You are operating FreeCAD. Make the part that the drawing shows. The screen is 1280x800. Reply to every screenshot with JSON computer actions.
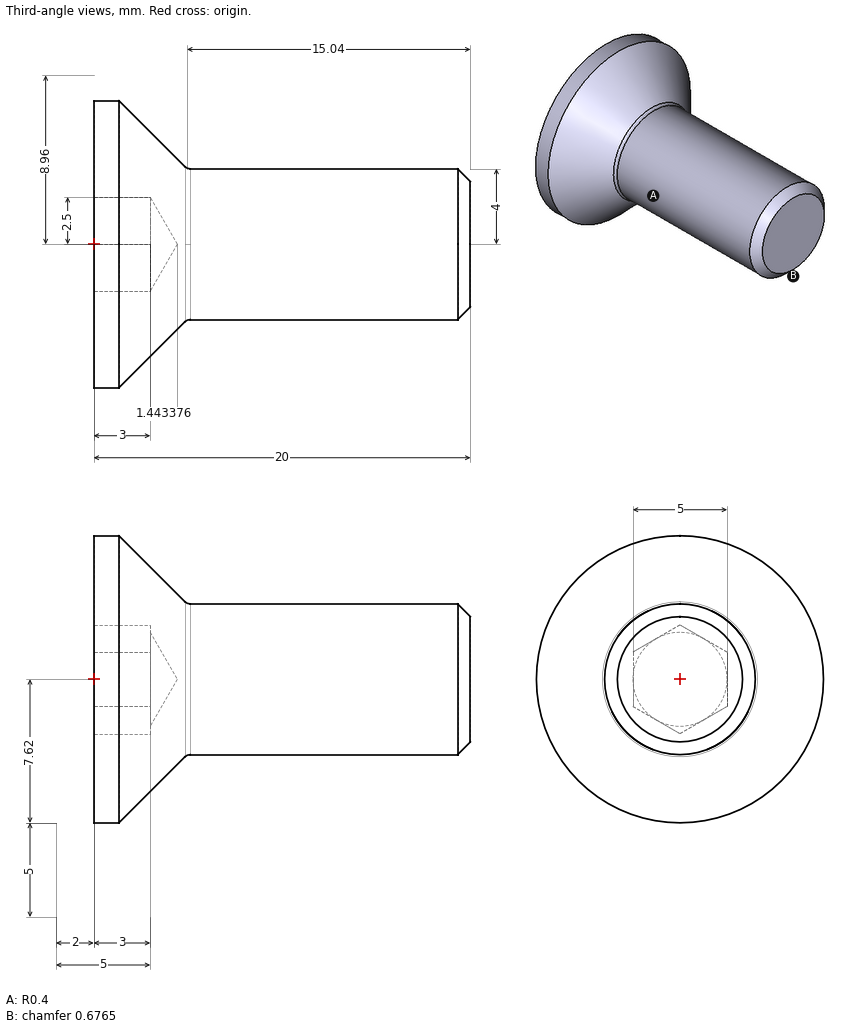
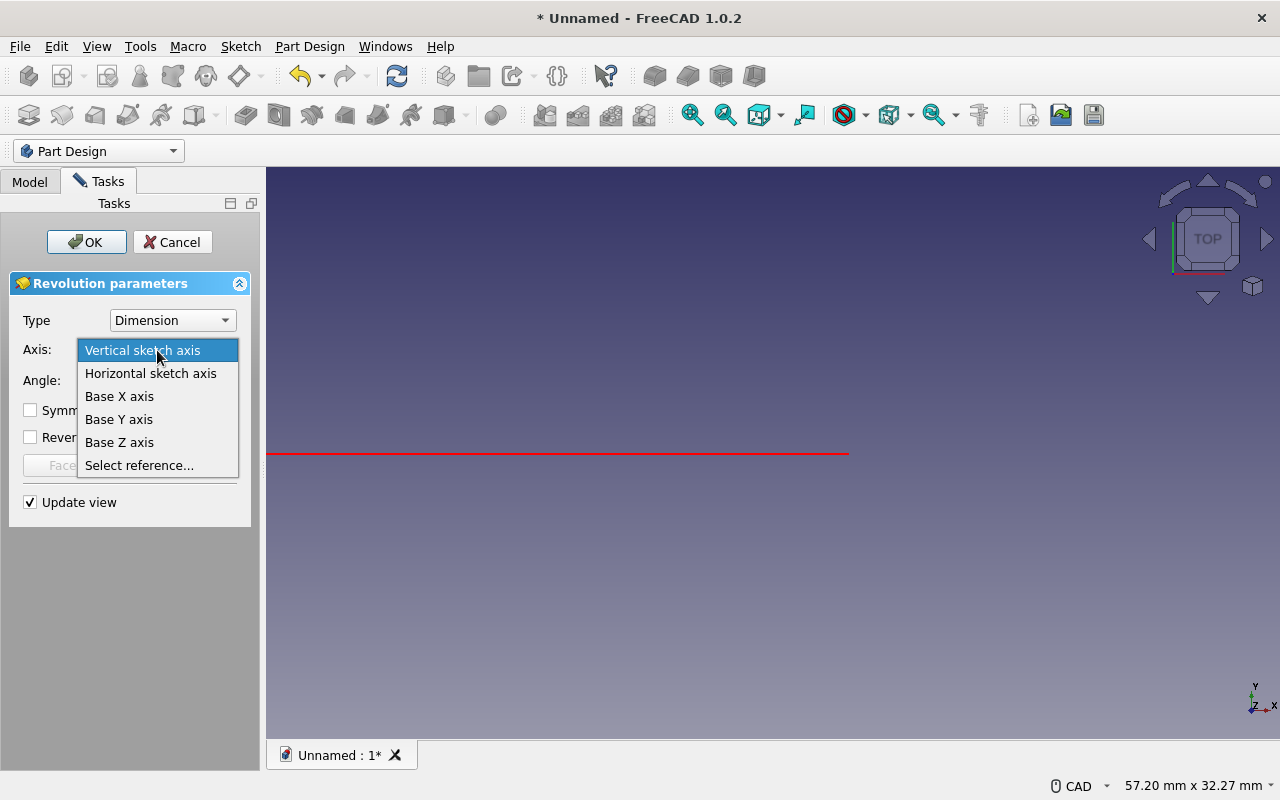
{"action": "left_click", "coordinate": [156, 374]}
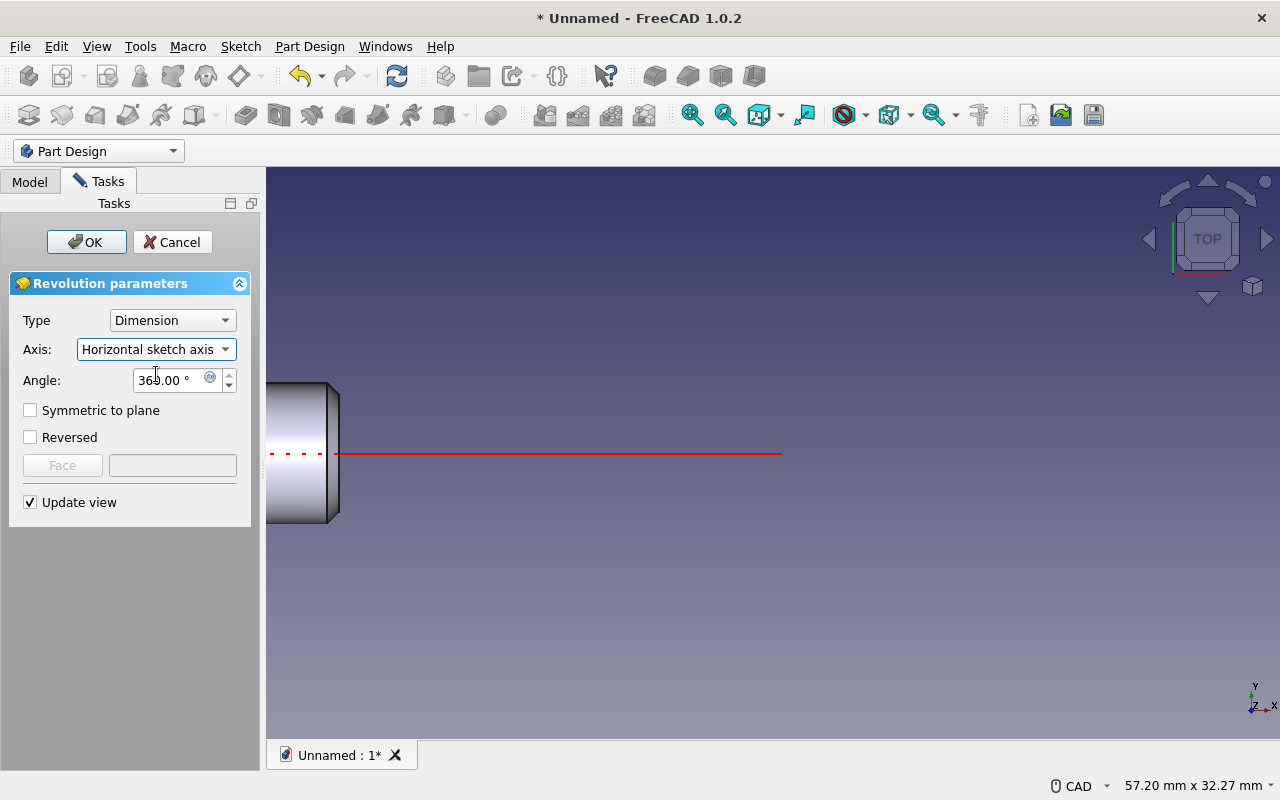
{"action": "left_click", "coordinate": [87, 242]}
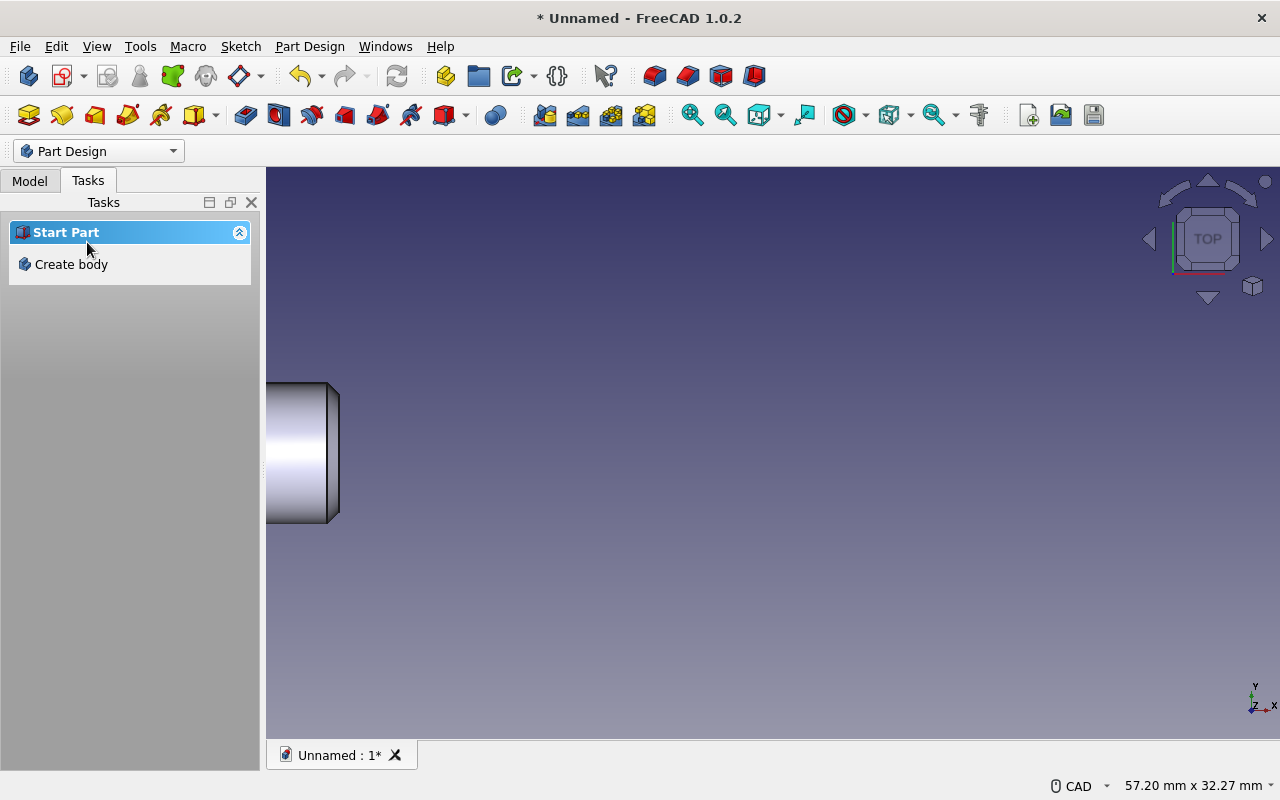
{"action": "key", "text": "0"}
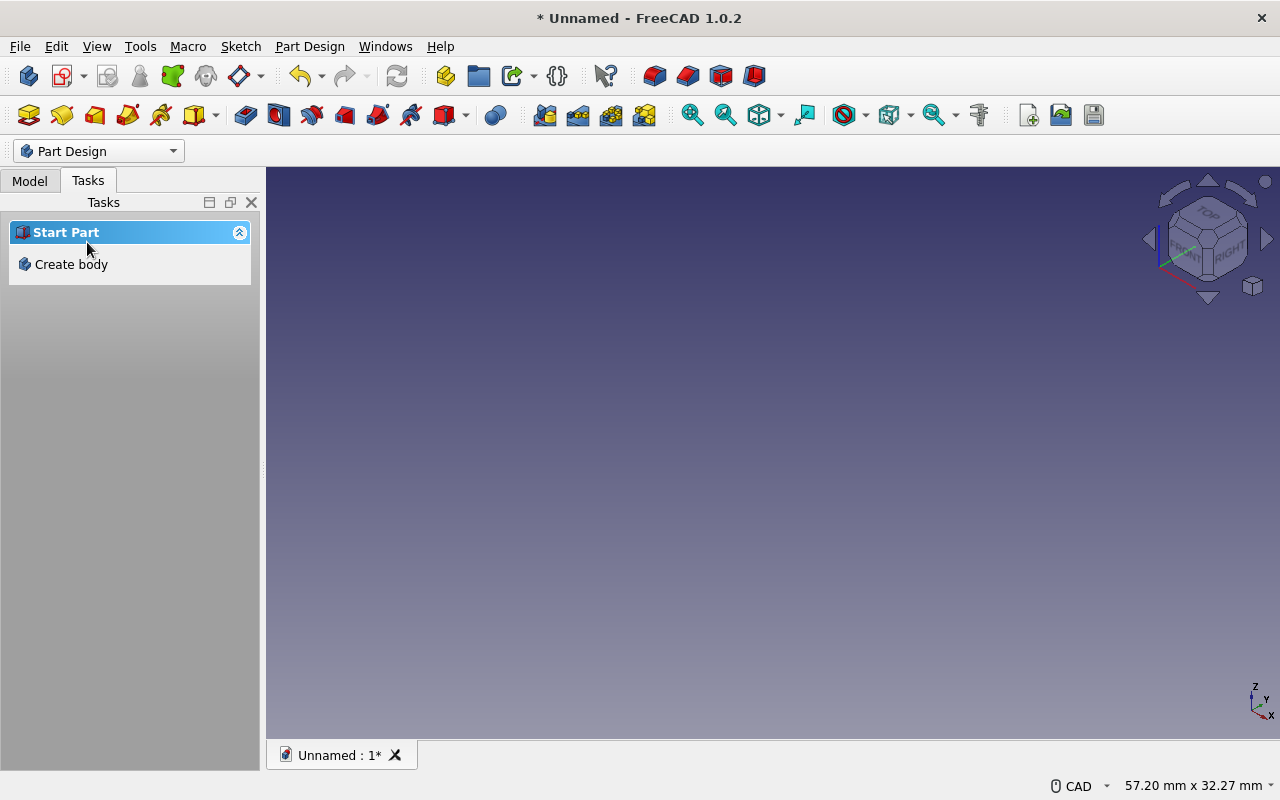
{"action": "left_click", "coordinate": [693, 116]}